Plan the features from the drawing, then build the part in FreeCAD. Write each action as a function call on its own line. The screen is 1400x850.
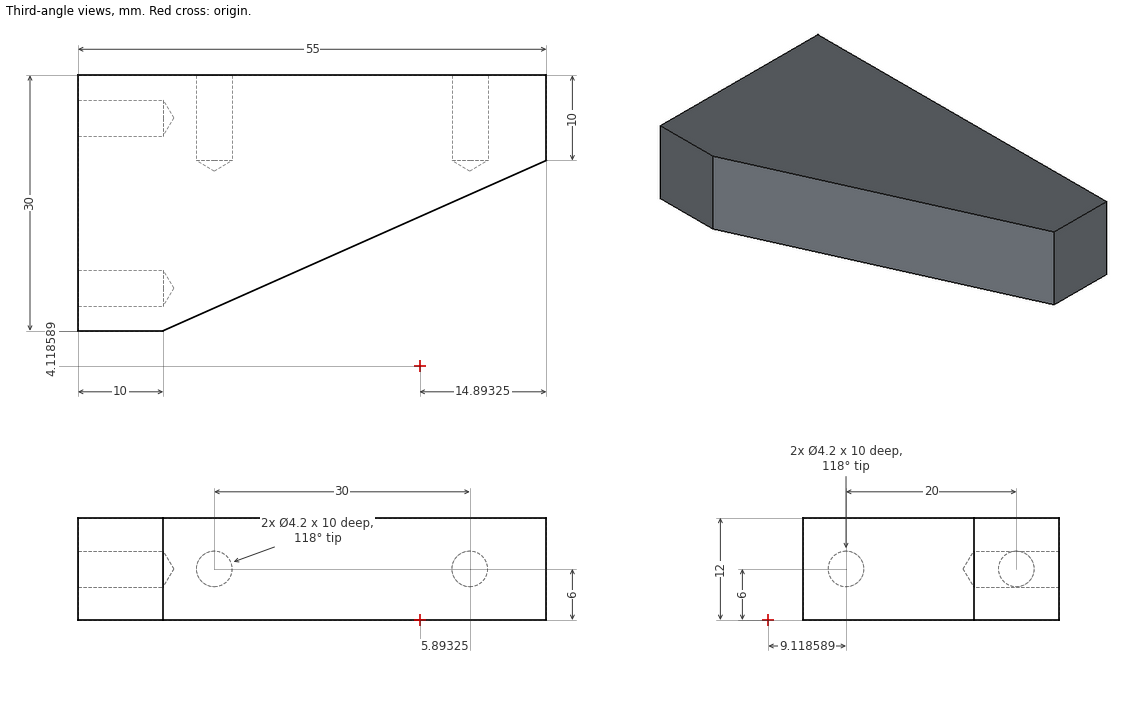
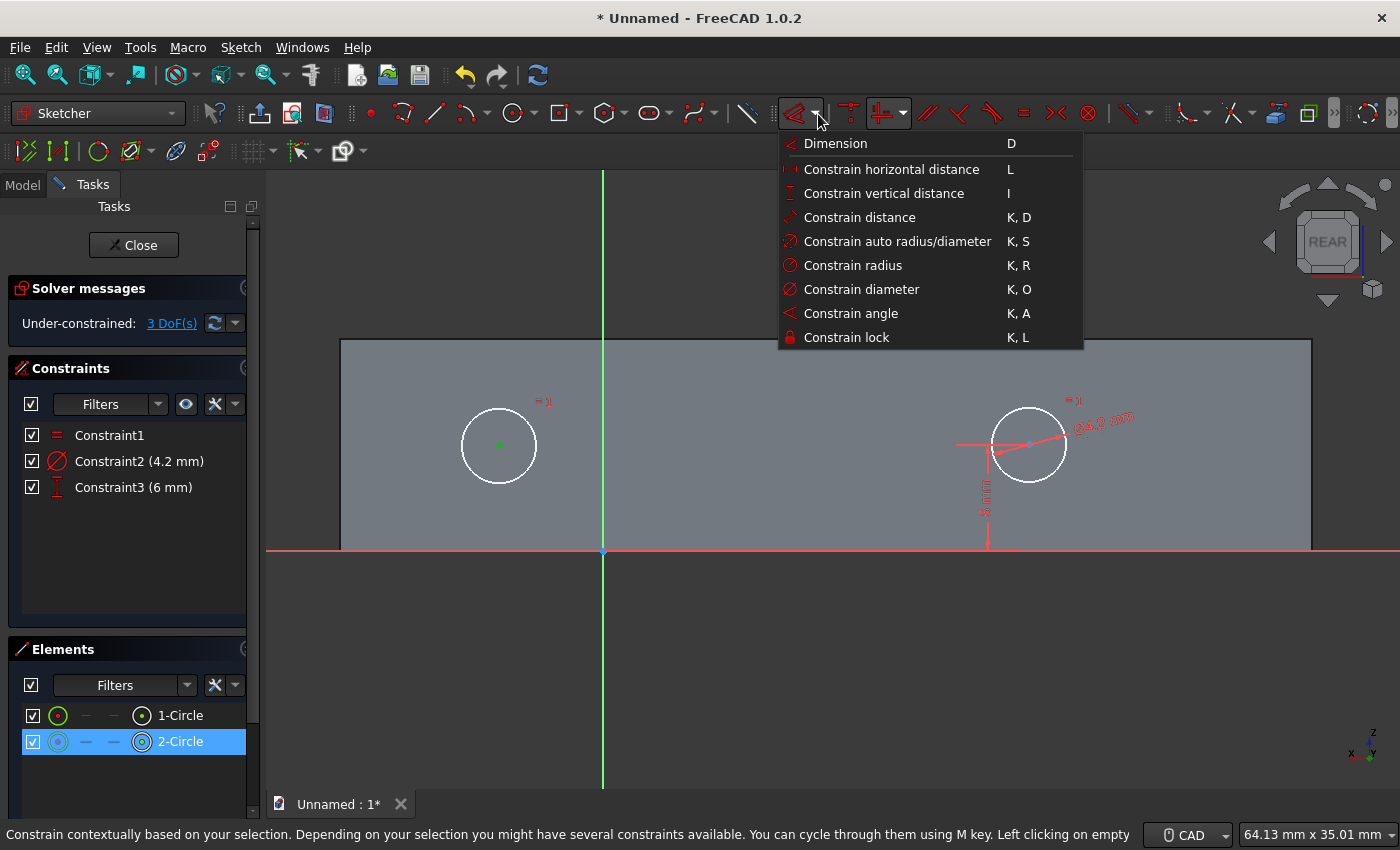
click(931, 193)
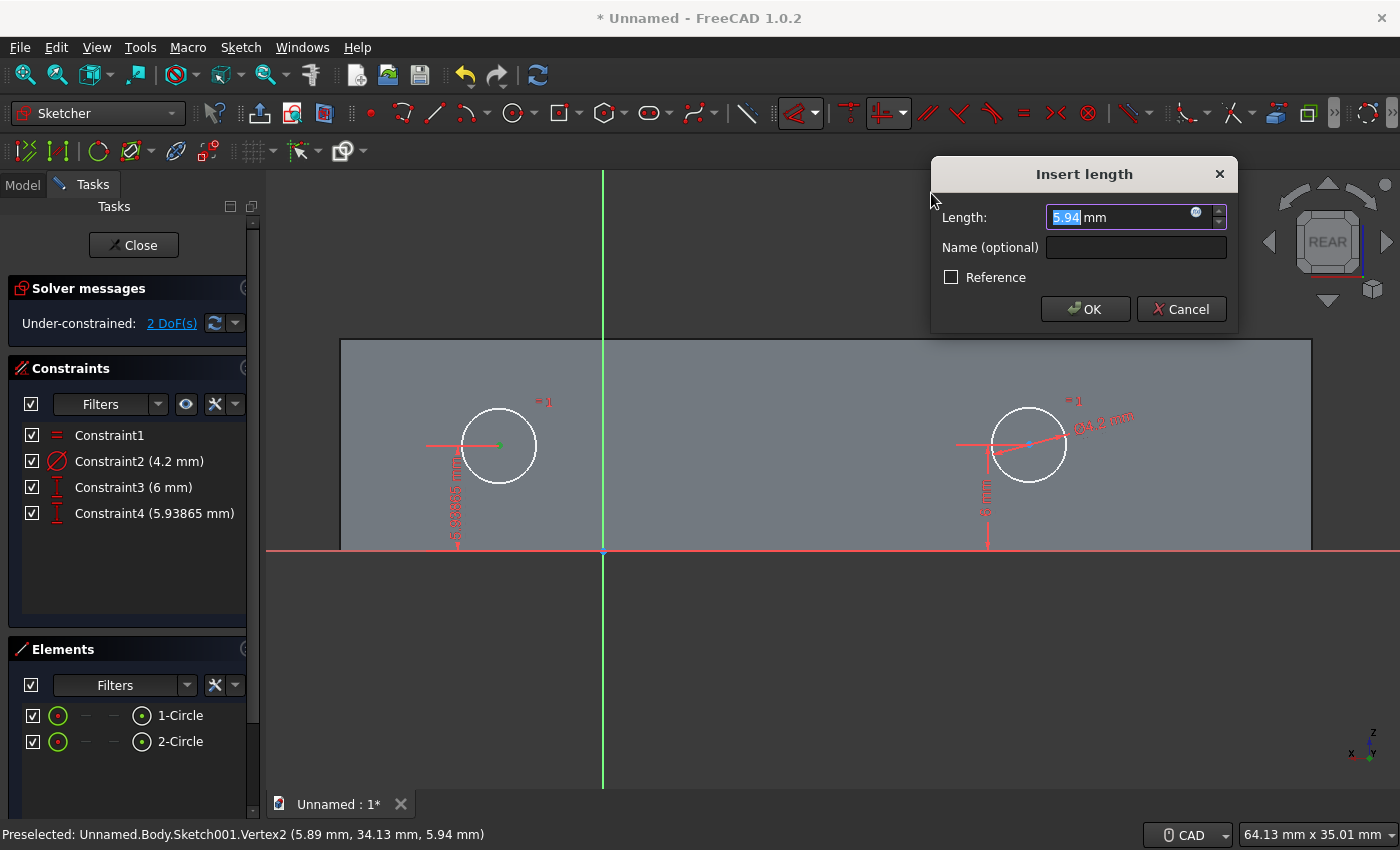
text(6)
key(Return)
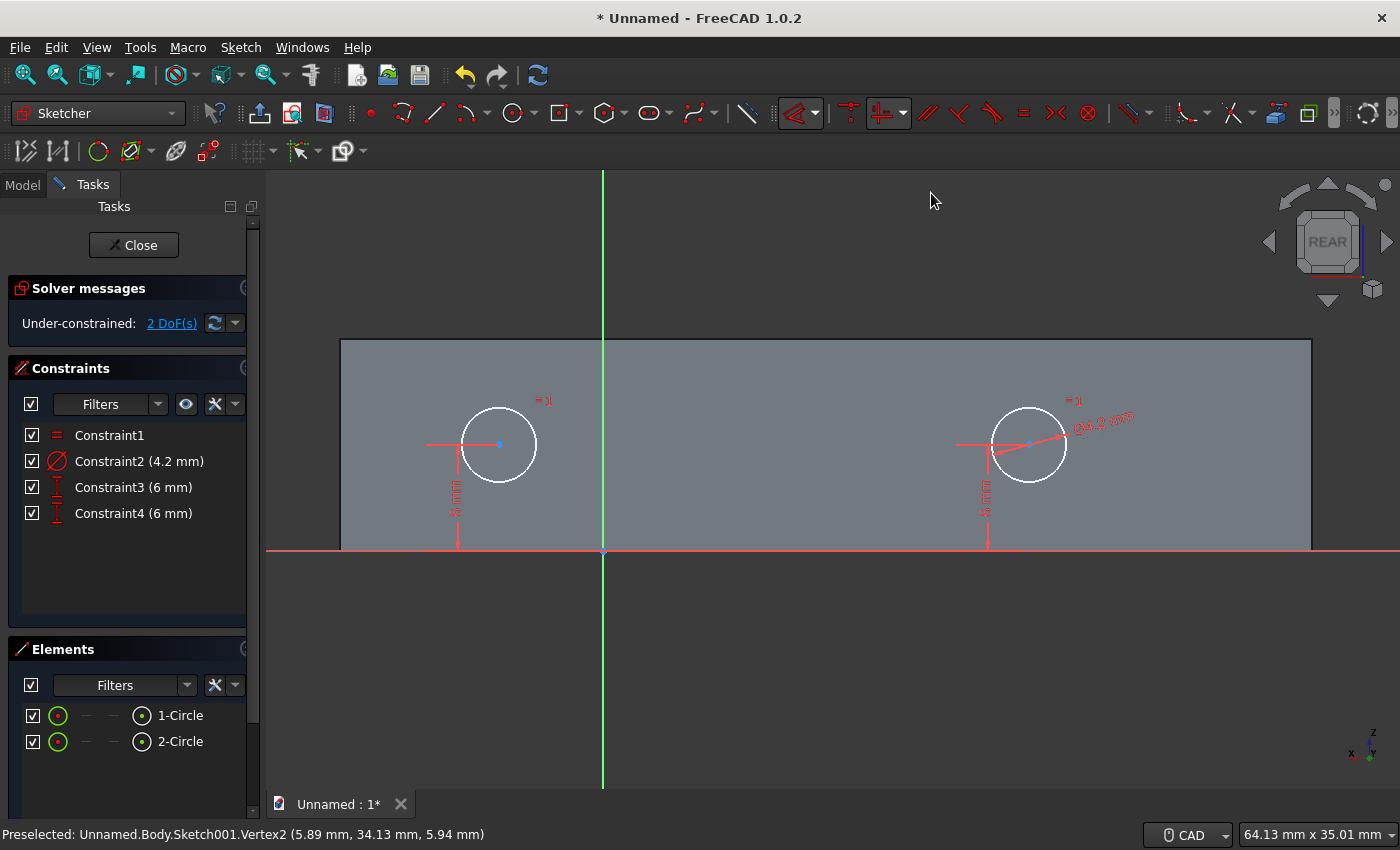
click(1029, 445)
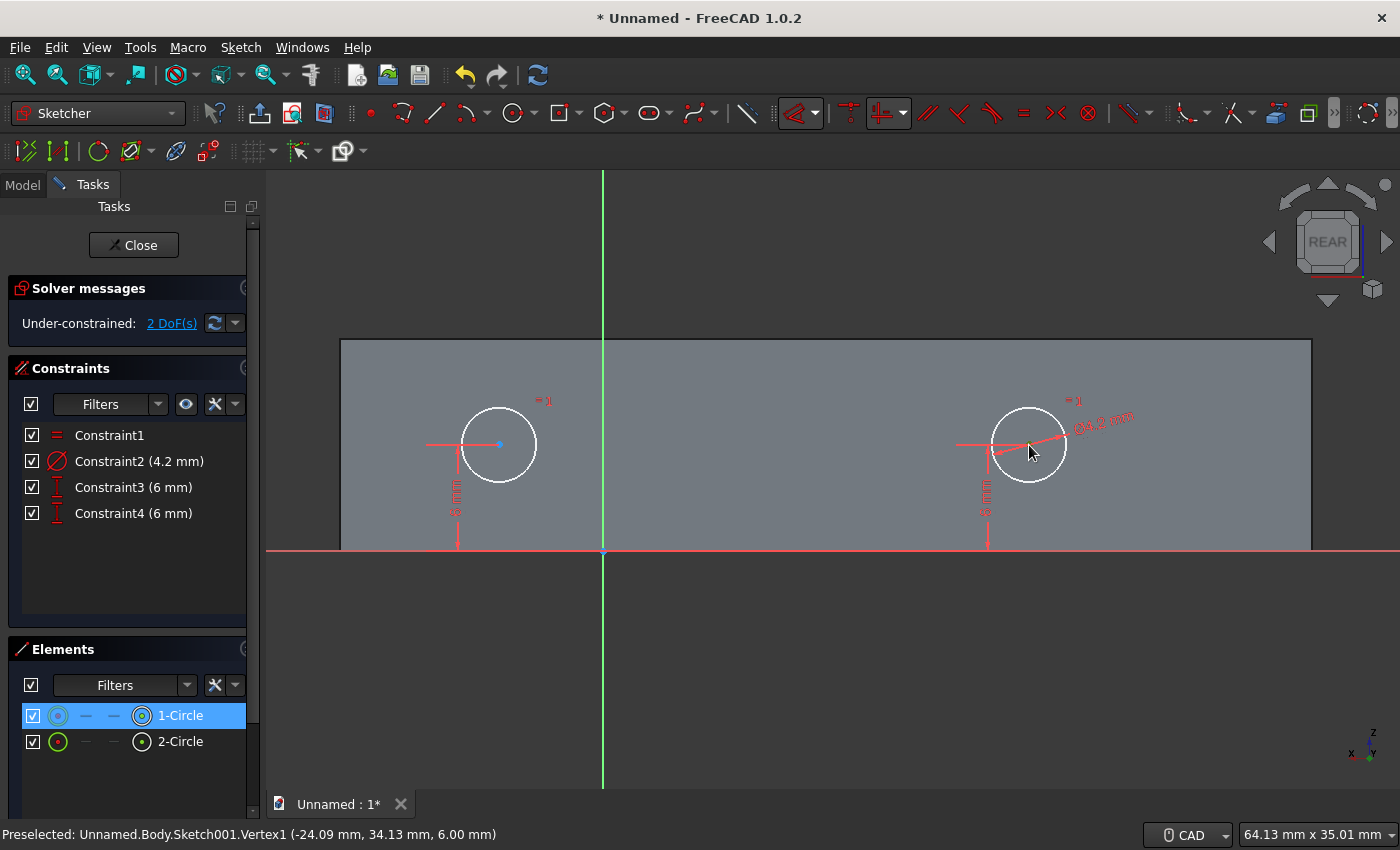
click(499, 445)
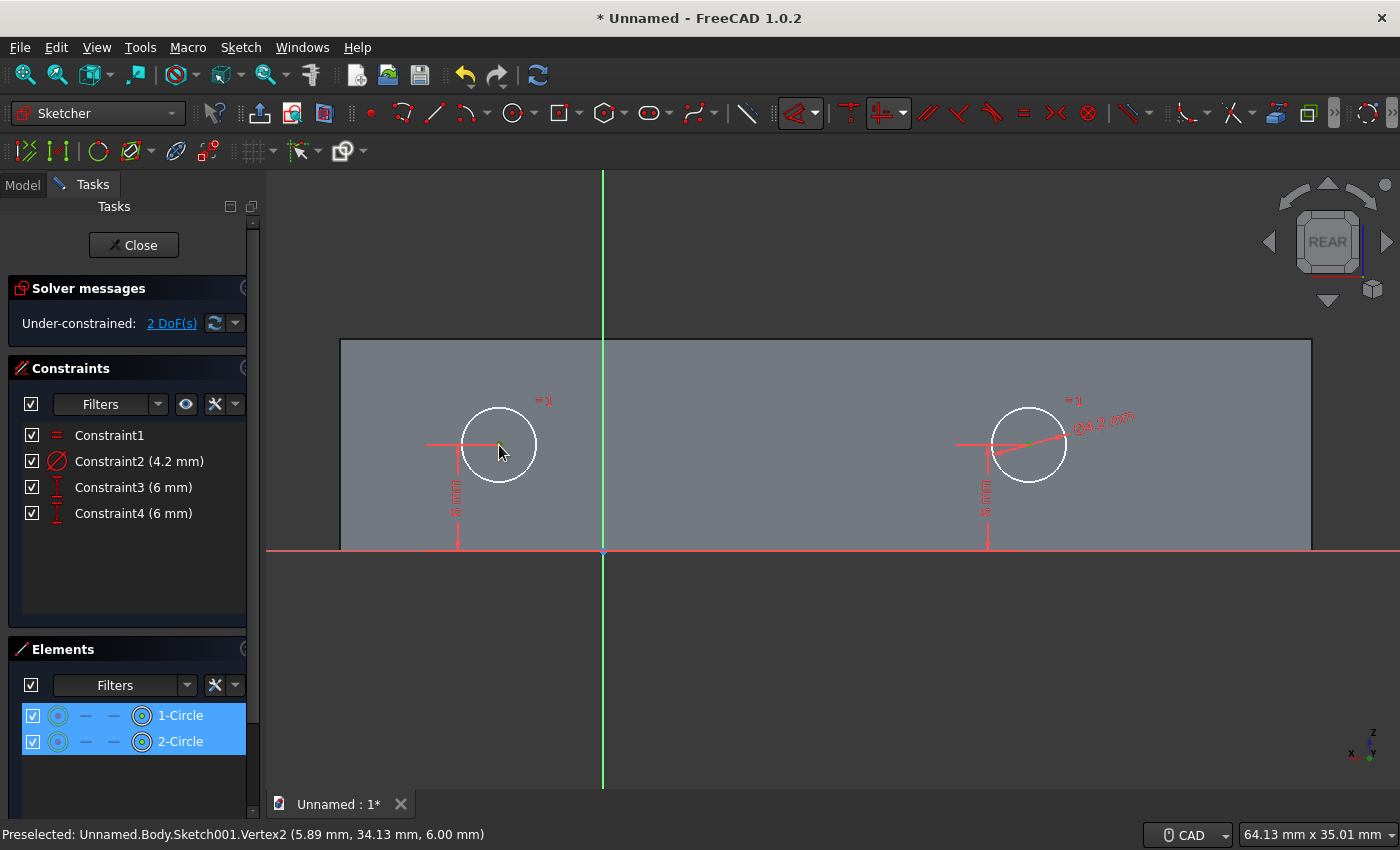
key(l)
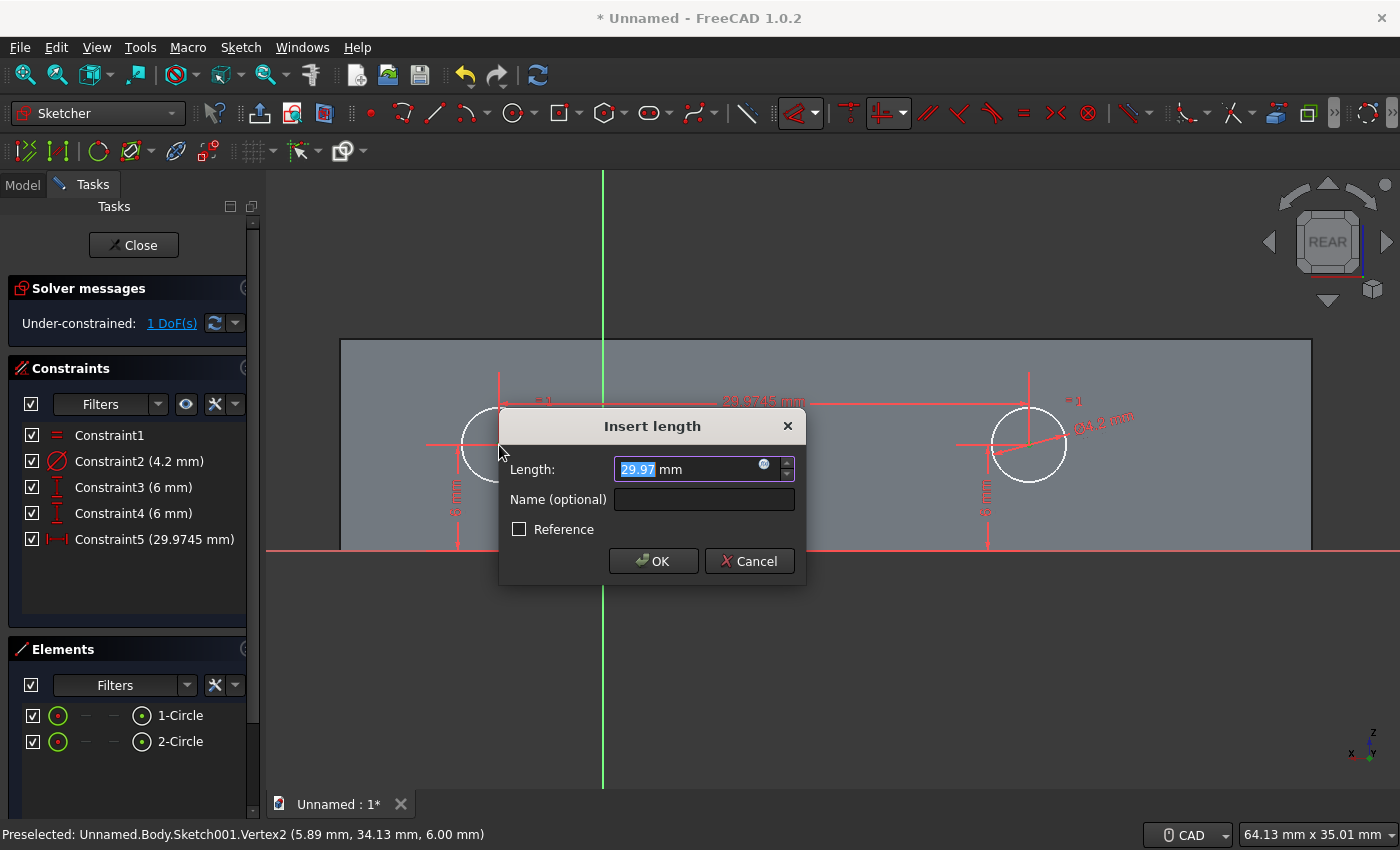
text(30)
key(Return)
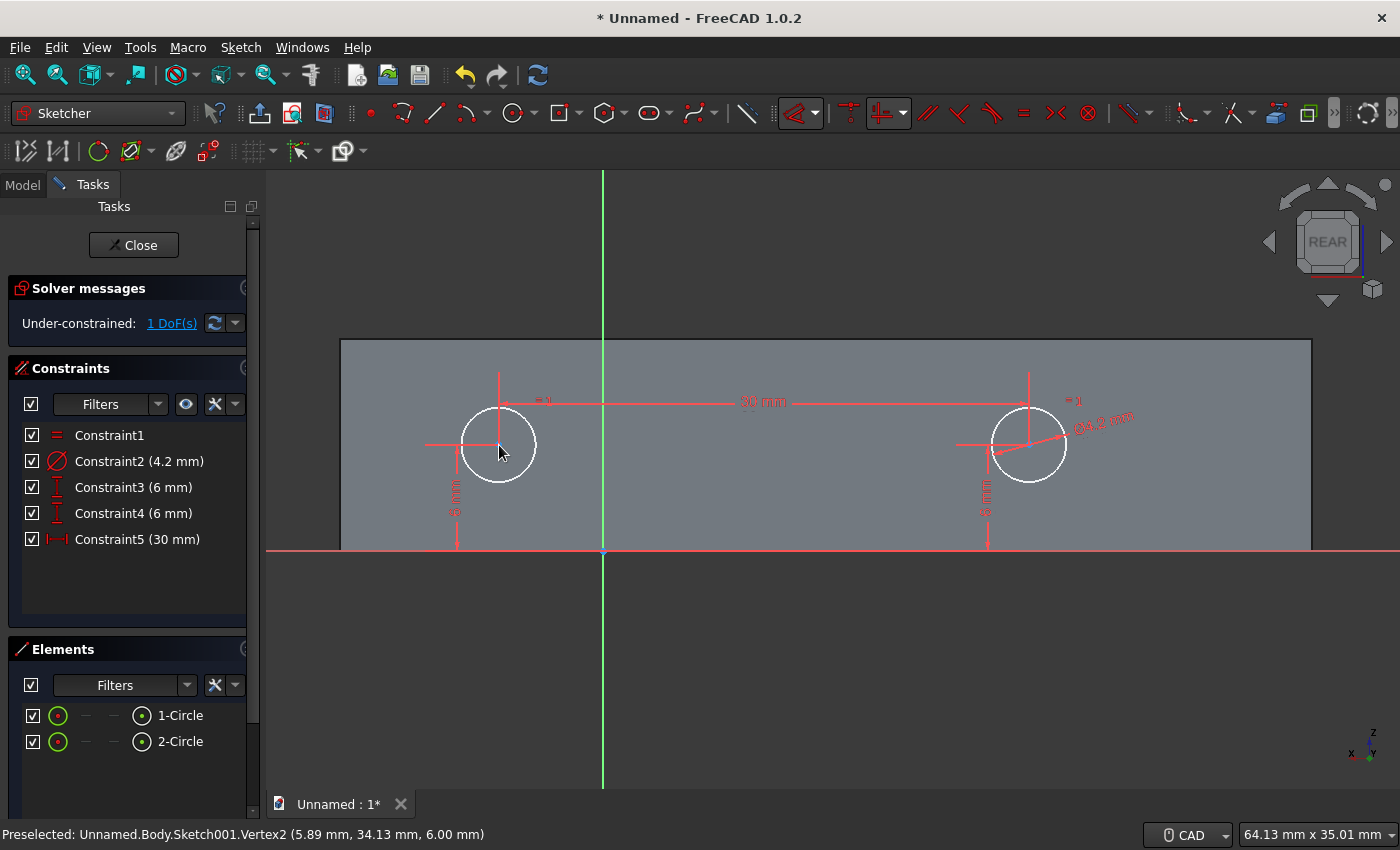
click(499, 445)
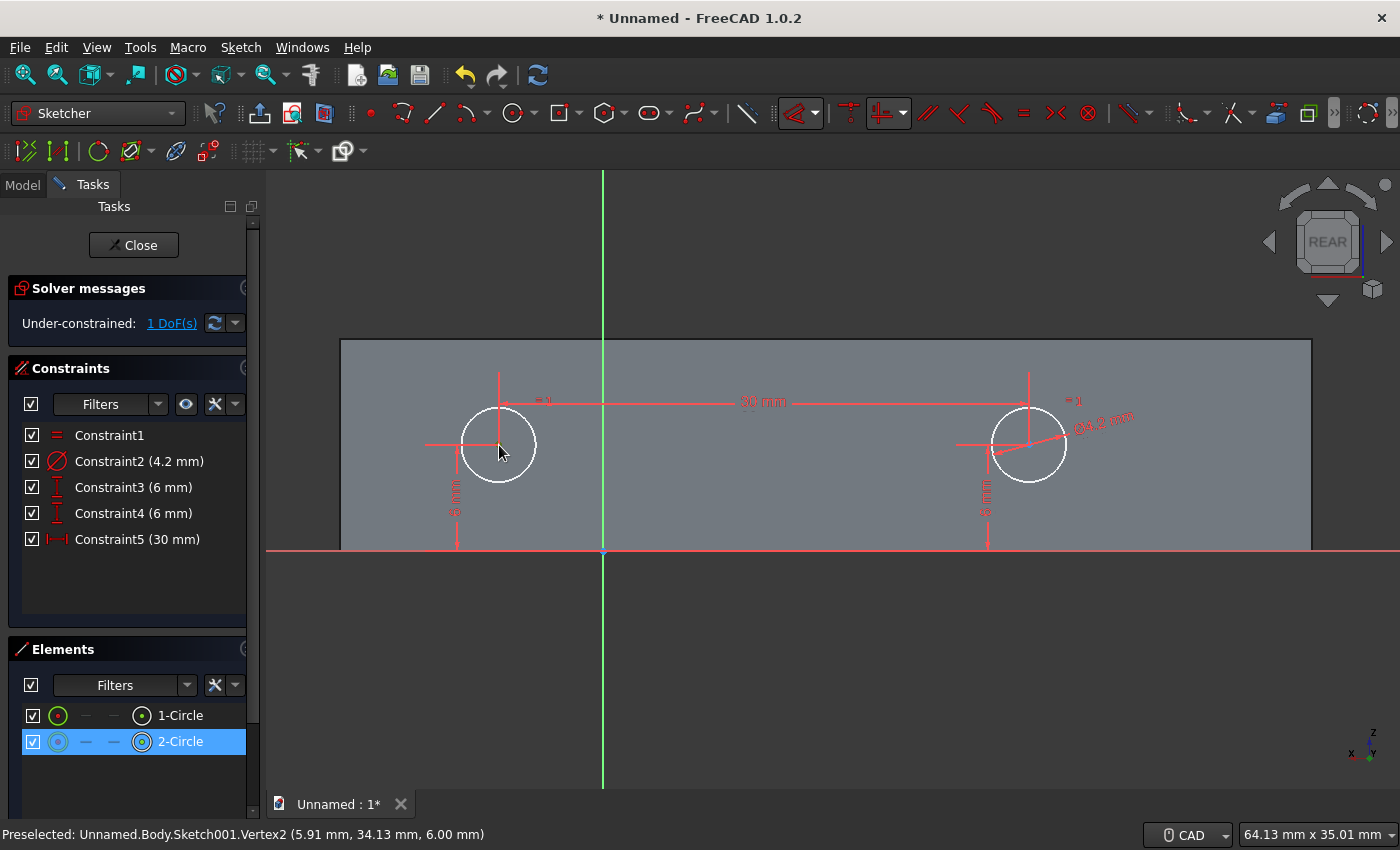
click(818, 114)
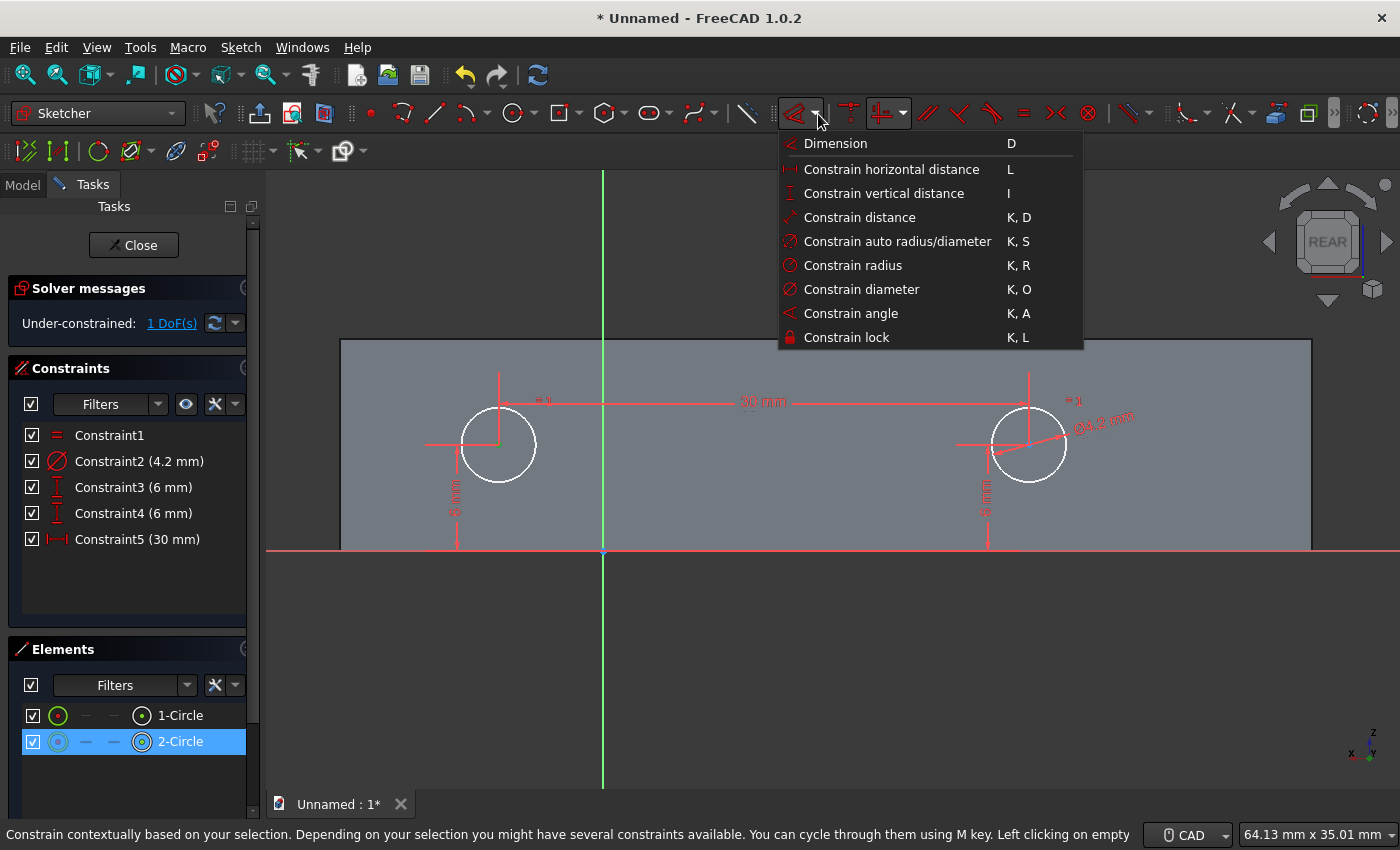
click(931, 169)